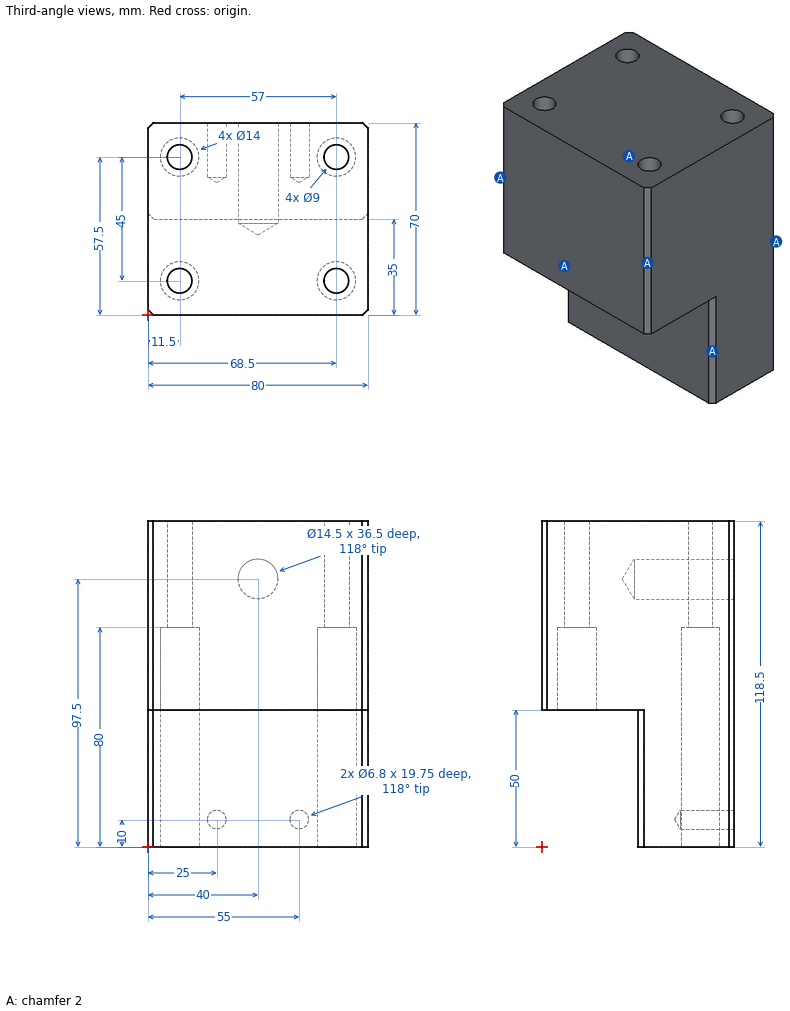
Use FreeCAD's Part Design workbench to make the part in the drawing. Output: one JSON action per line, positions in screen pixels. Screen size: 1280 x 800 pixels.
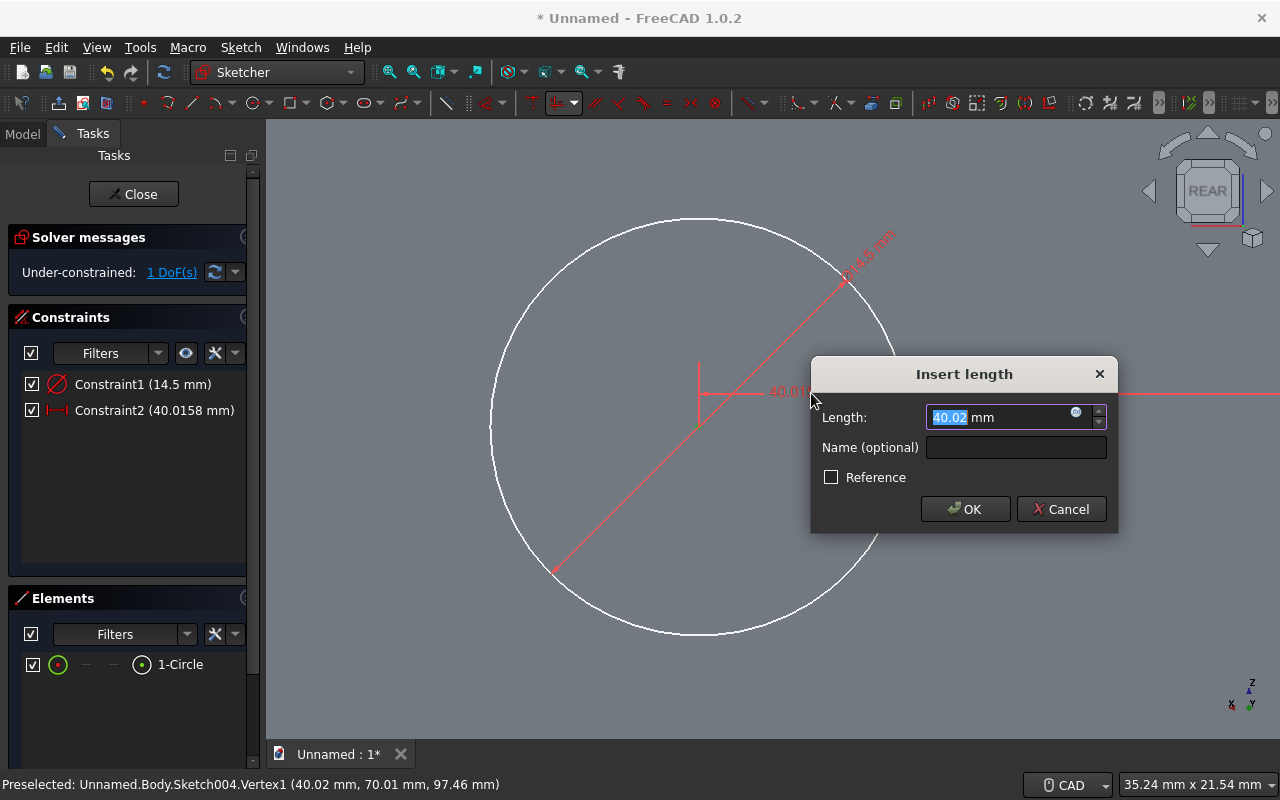
{"action": "type", "text": "40"}
{"action": "key", "text": "Return"}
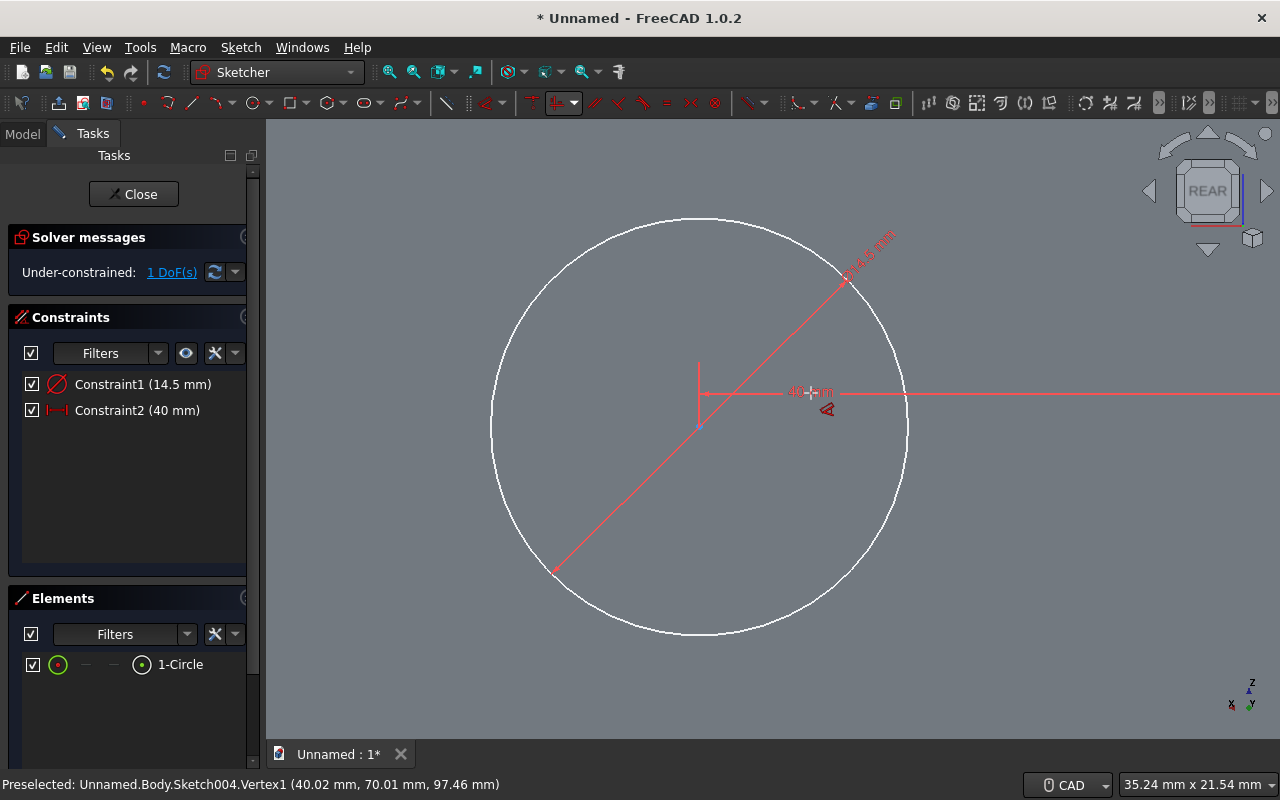
{"action": "left_click", "coordinate": [699, 427]}
{"action": "left_click", "coordinate": [665, 569]}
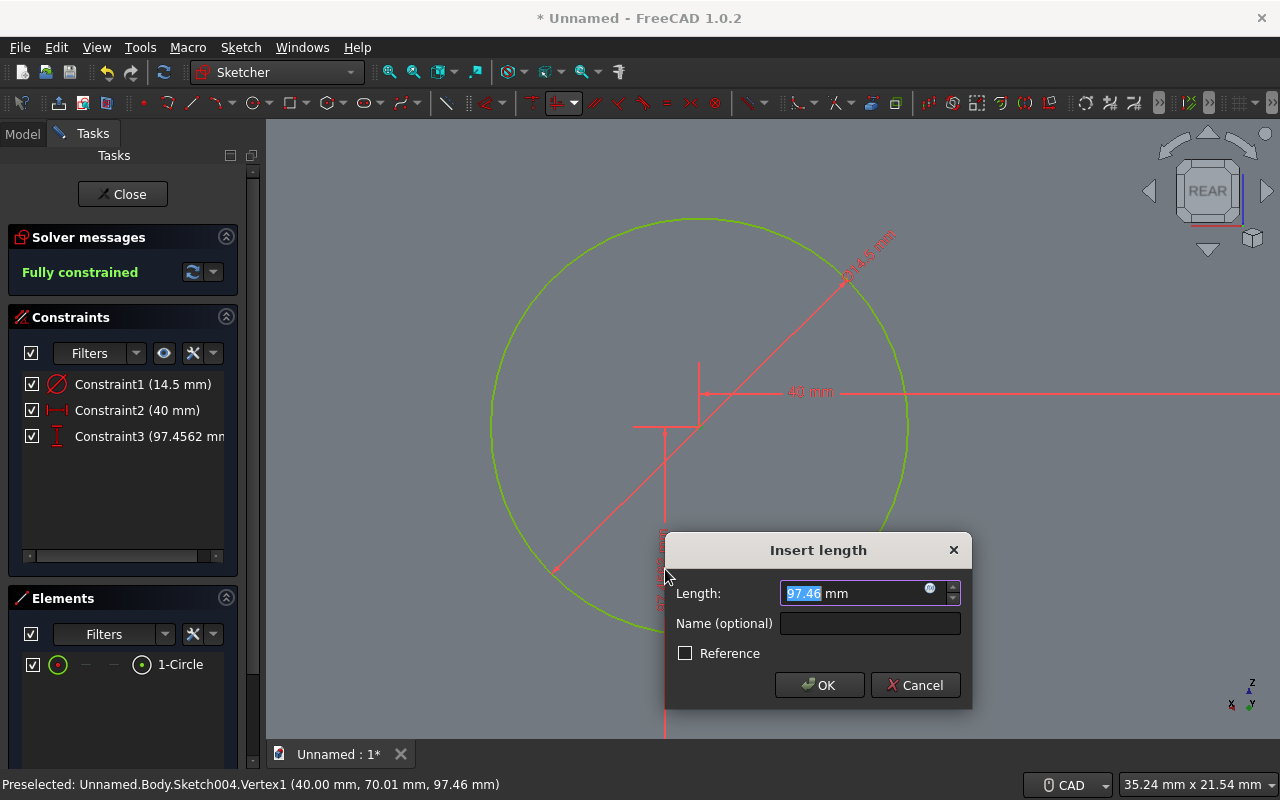
{"action": "type", "text": "97.5"}
{"action": "key", "text": "Return"}
{"action": "key", "text": "Escape"}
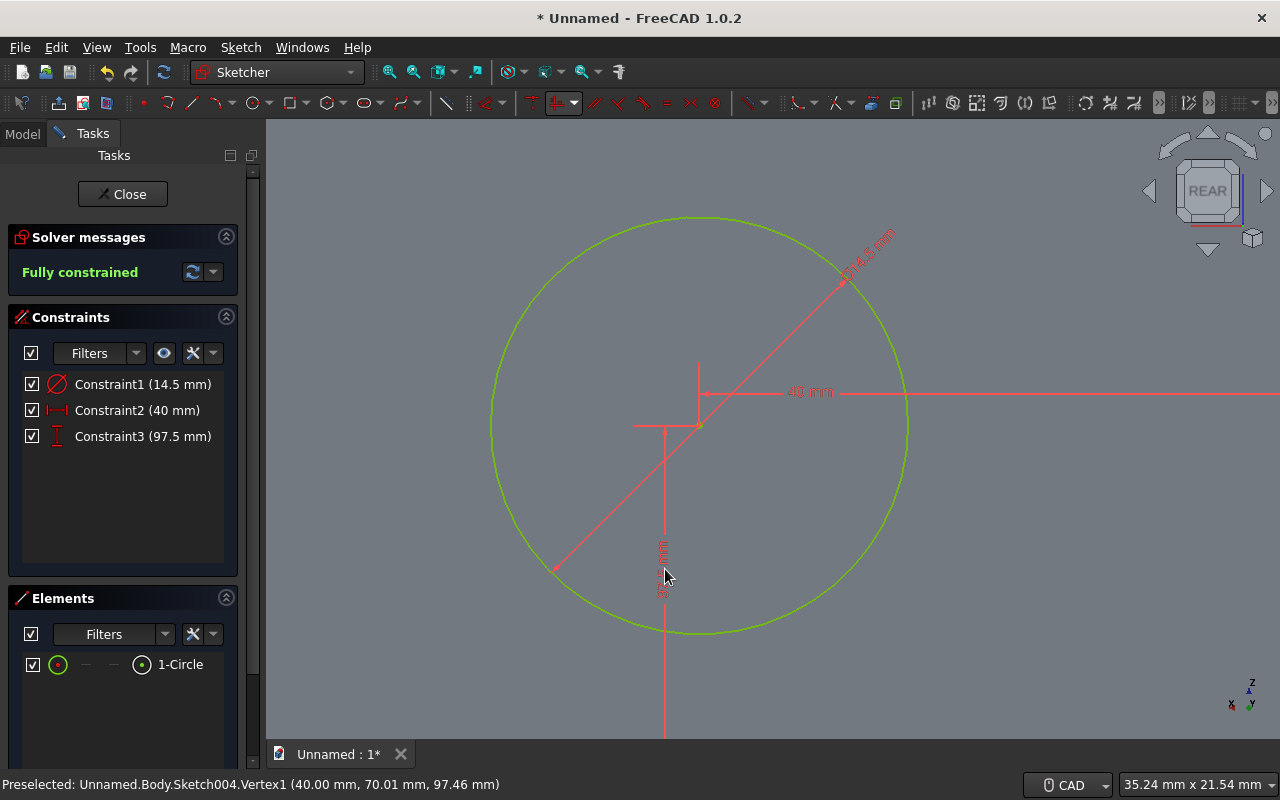
{"action": "left_click", "coordinate": [123, 194]}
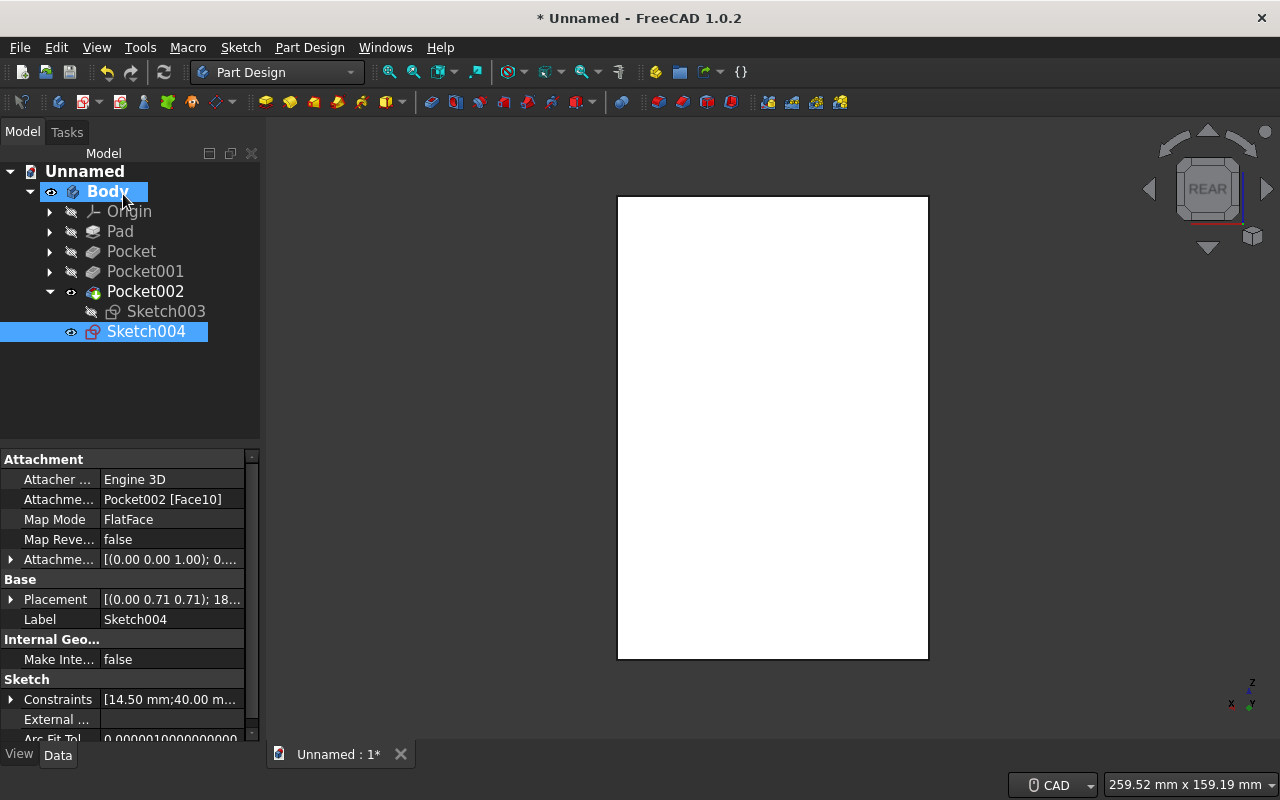
{"action": "left_click", "coordinate": [456, 102]}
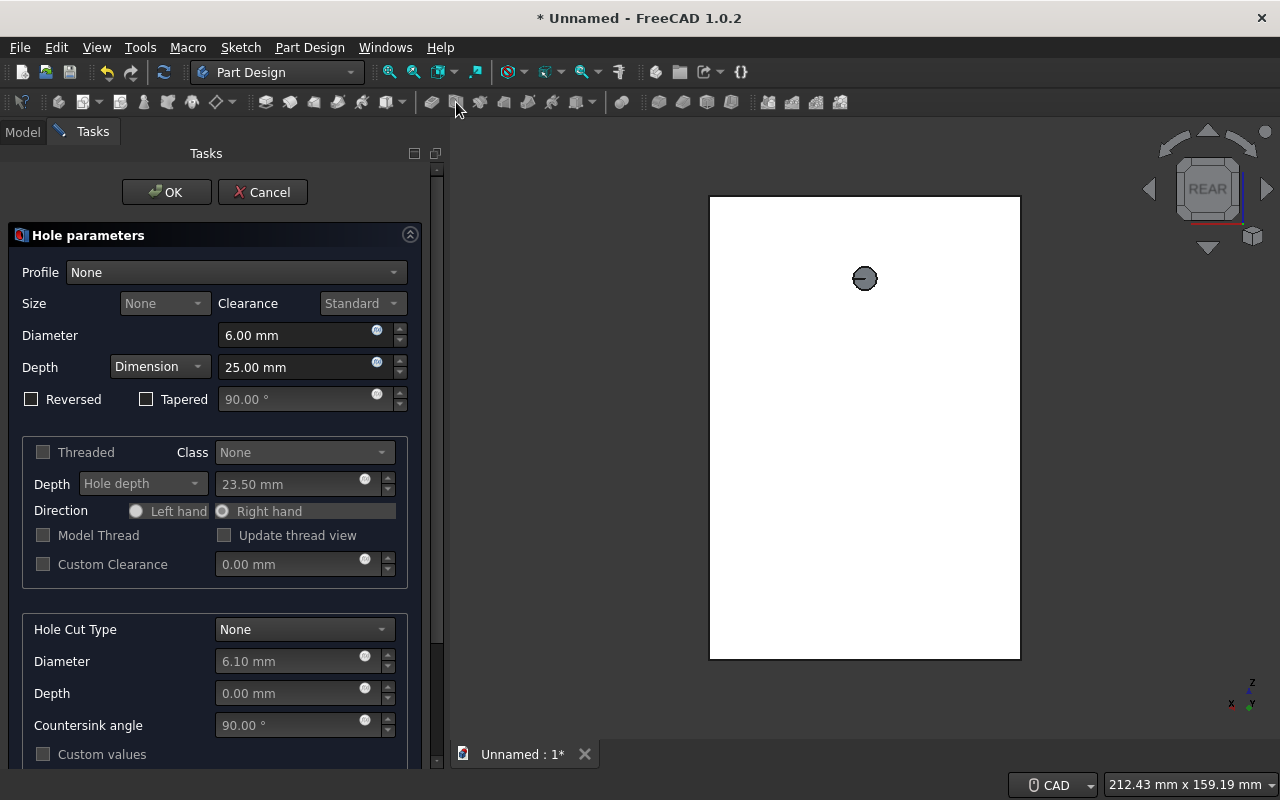
{"action": "triple_click", "coordinate": [305, 335]}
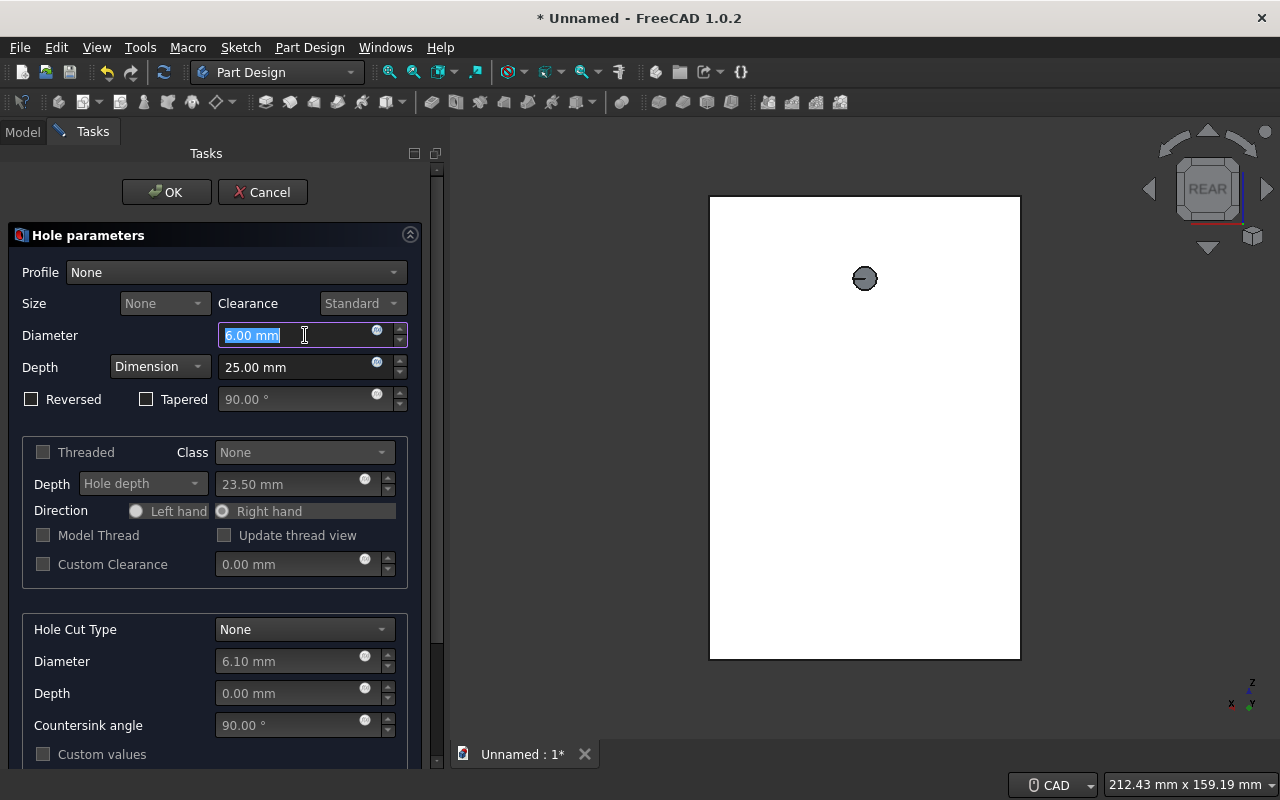
{"action": "type", "text": "14.5"}
{"action": "key", "text": "Tab"}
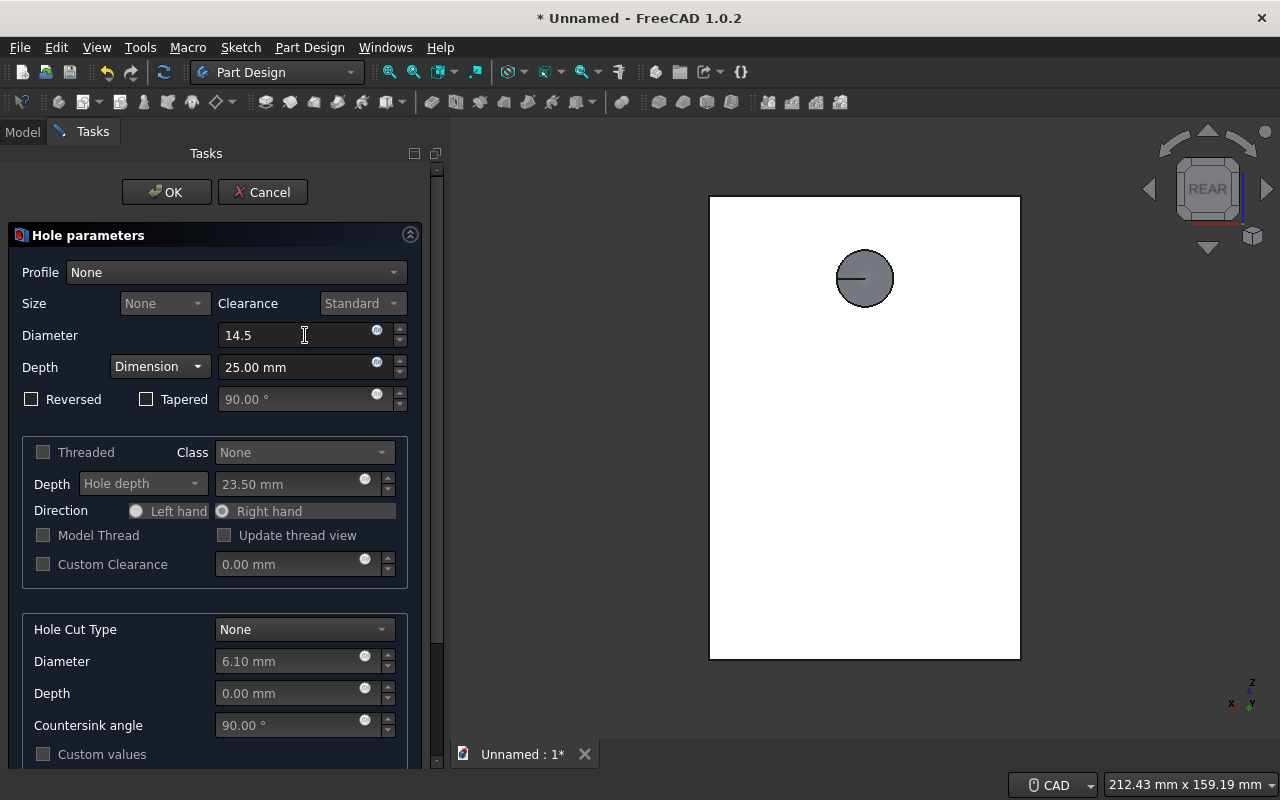
{"action": "triple_click", "coordinate": [305, 367]}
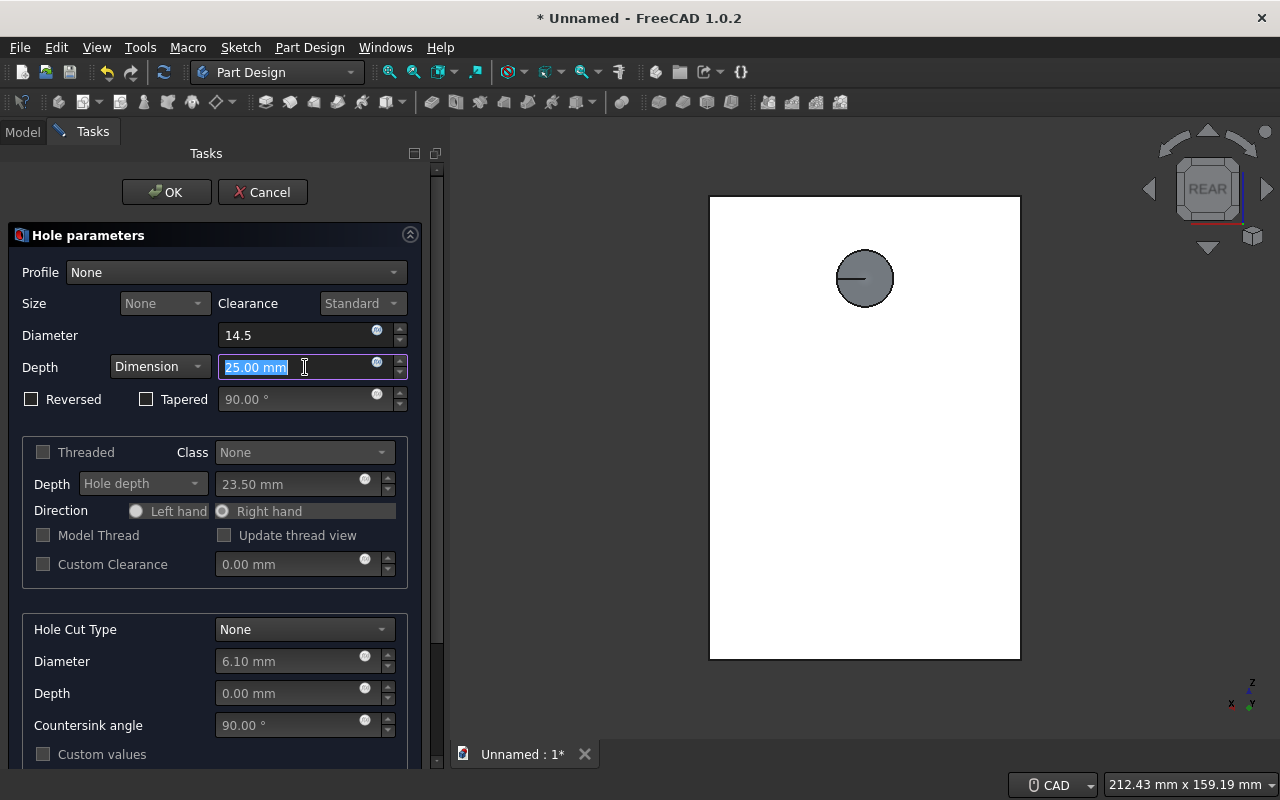
{"action": "type", "text": "36.5"}
{"action": "key", "text": "Tab"}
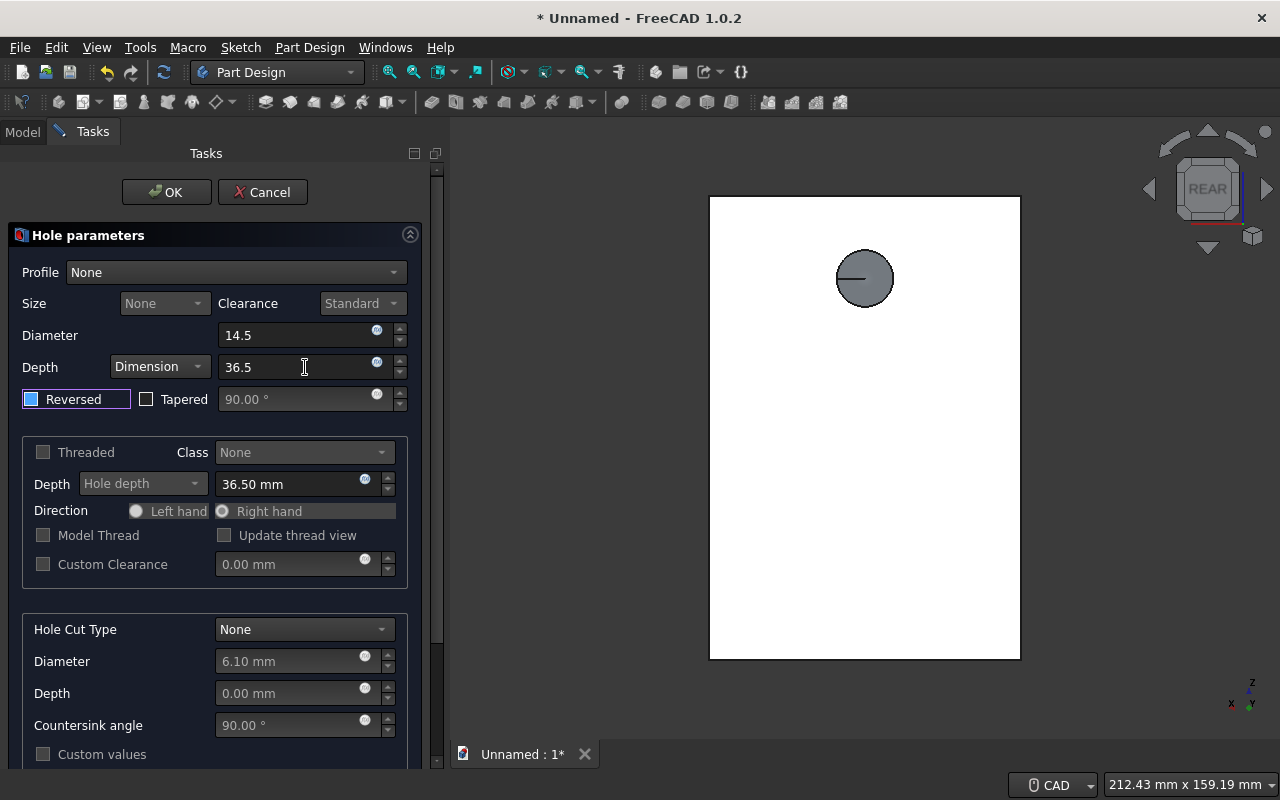
{"action": "left_click", "coordinate": [167, 192]}